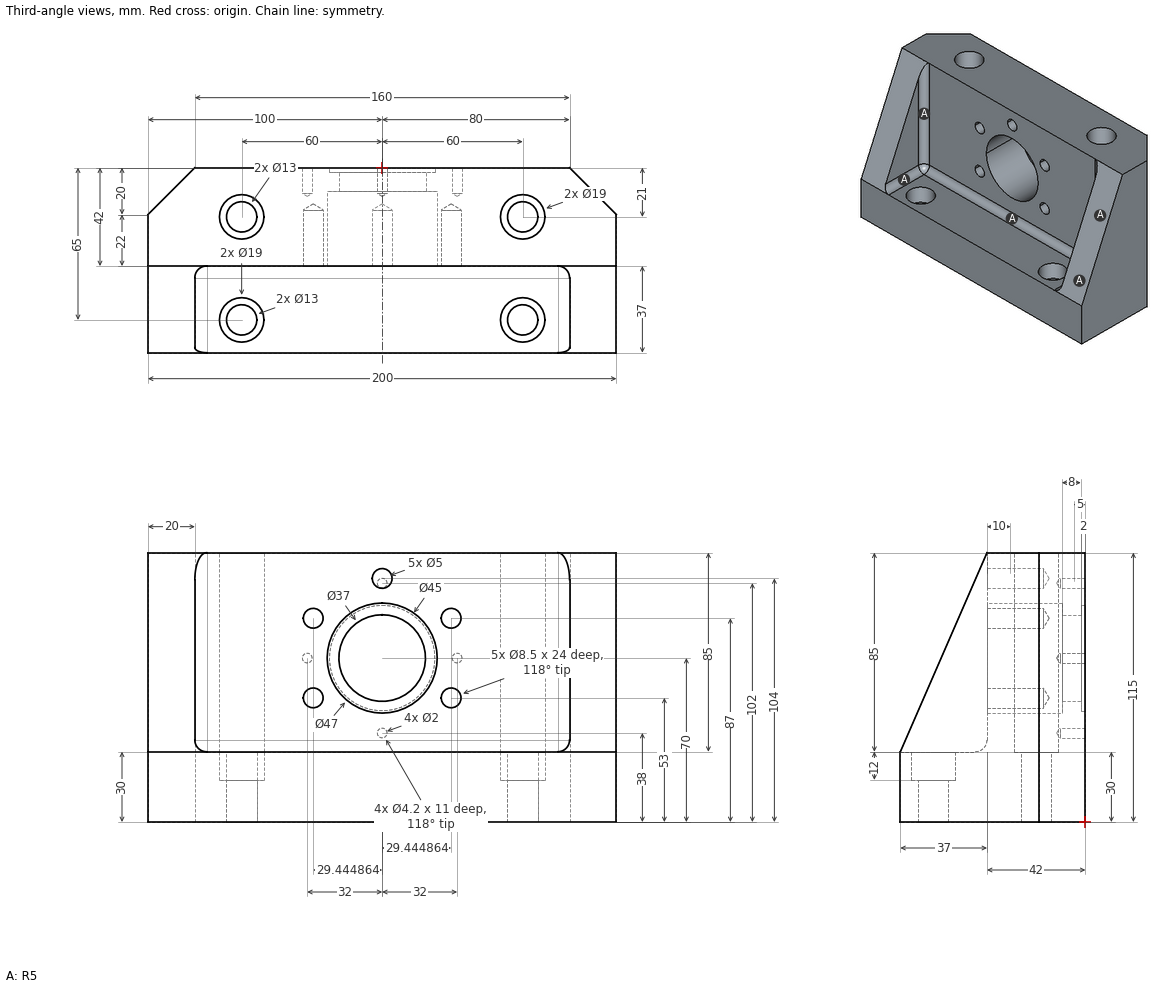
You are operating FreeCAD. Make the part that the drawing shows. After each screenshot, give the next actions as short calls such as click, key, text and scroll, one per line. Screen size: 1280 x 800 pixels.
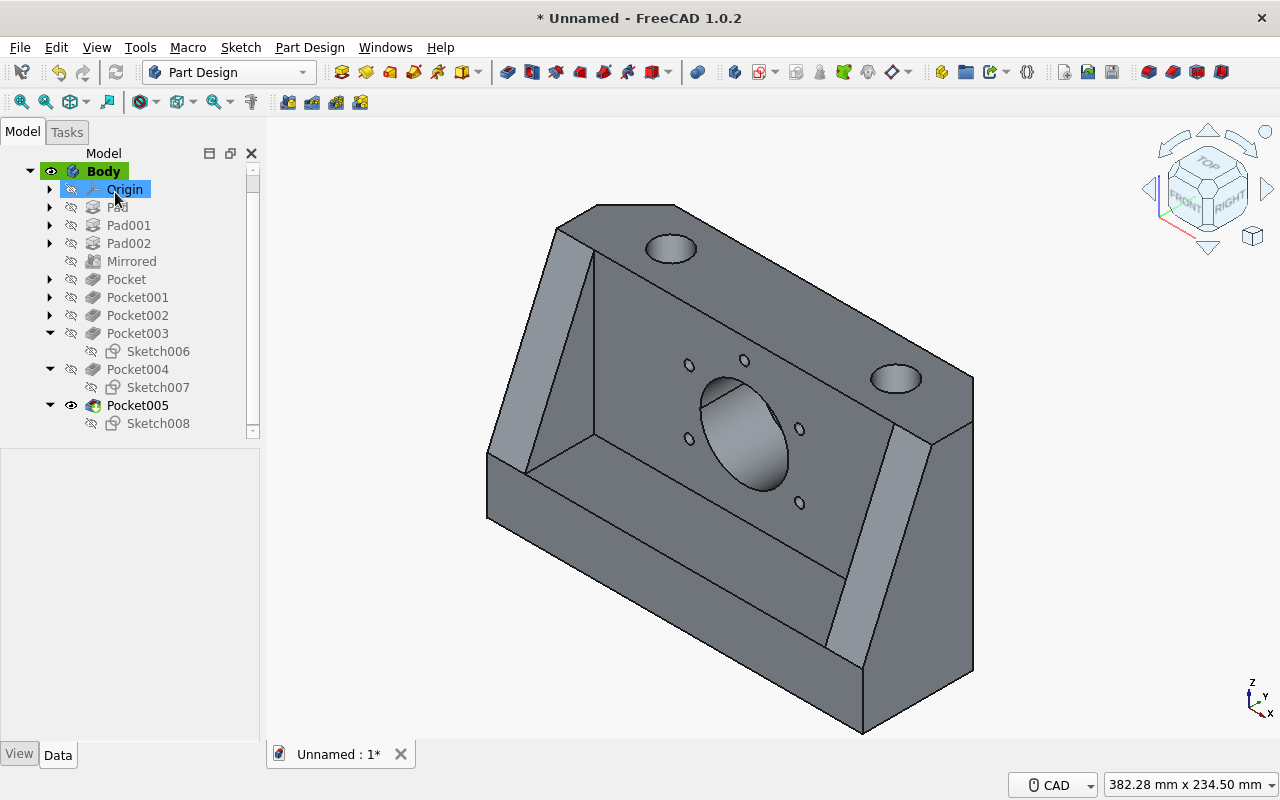
key(2)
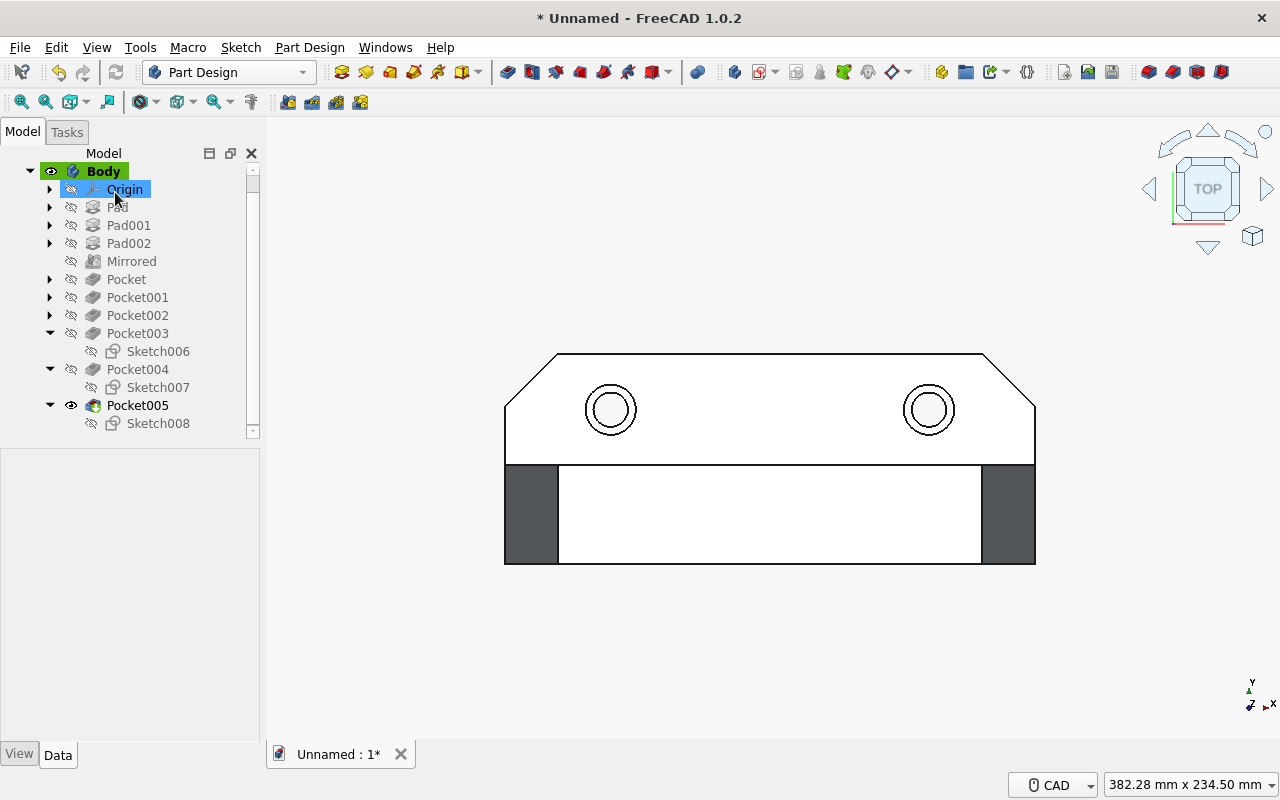
key(0)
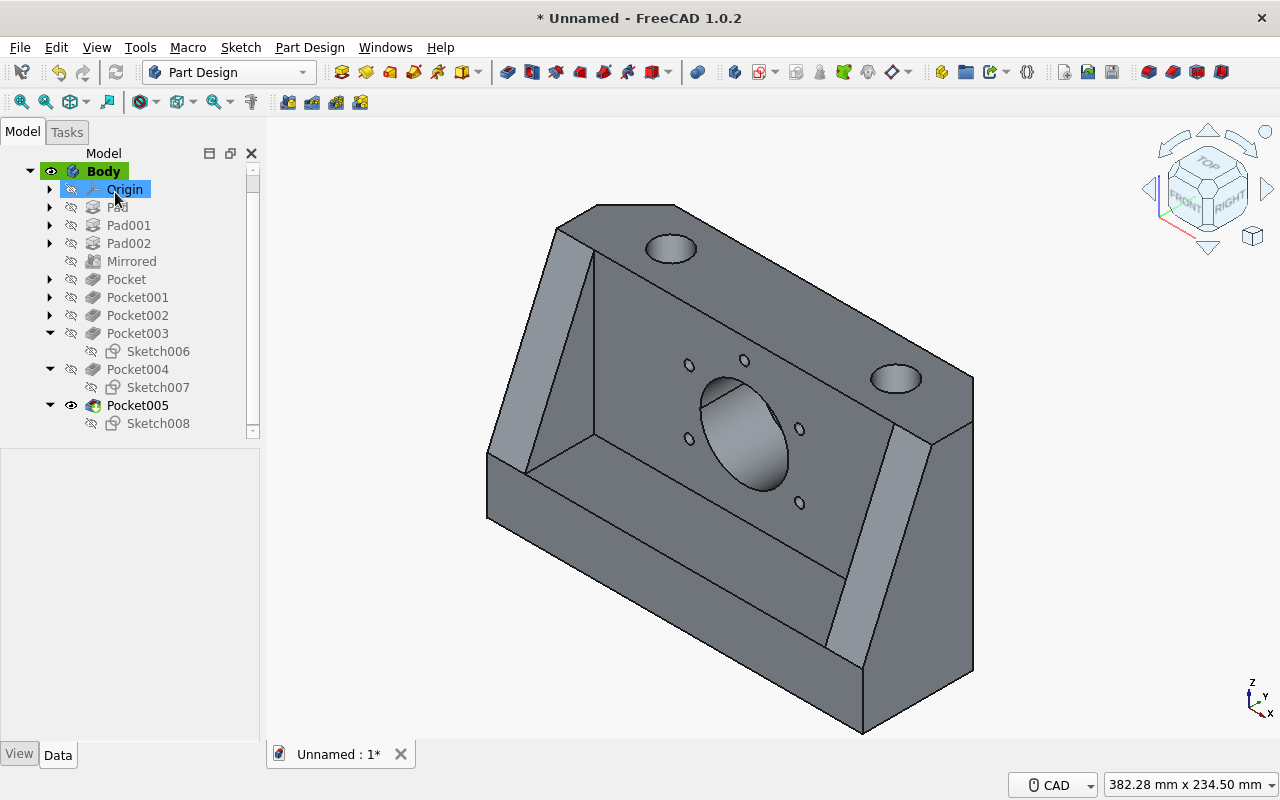
key(1)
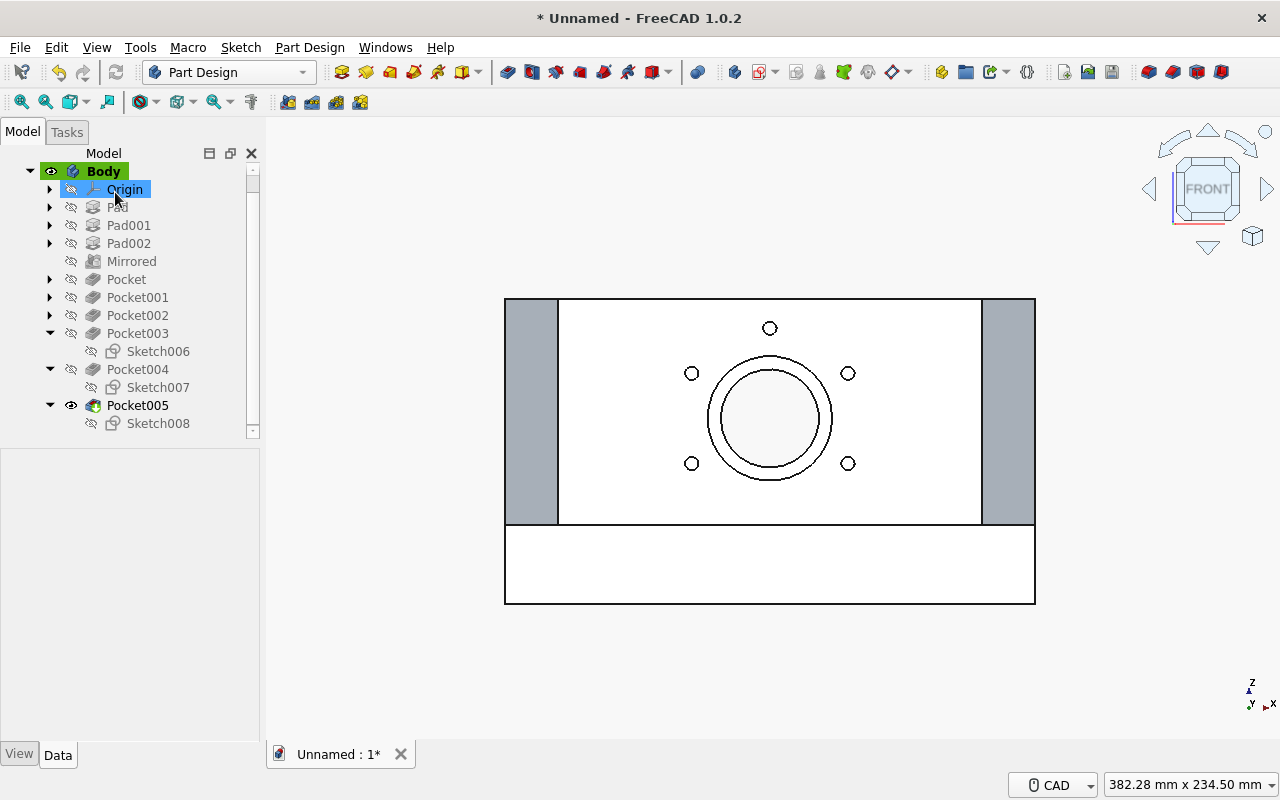
key(3)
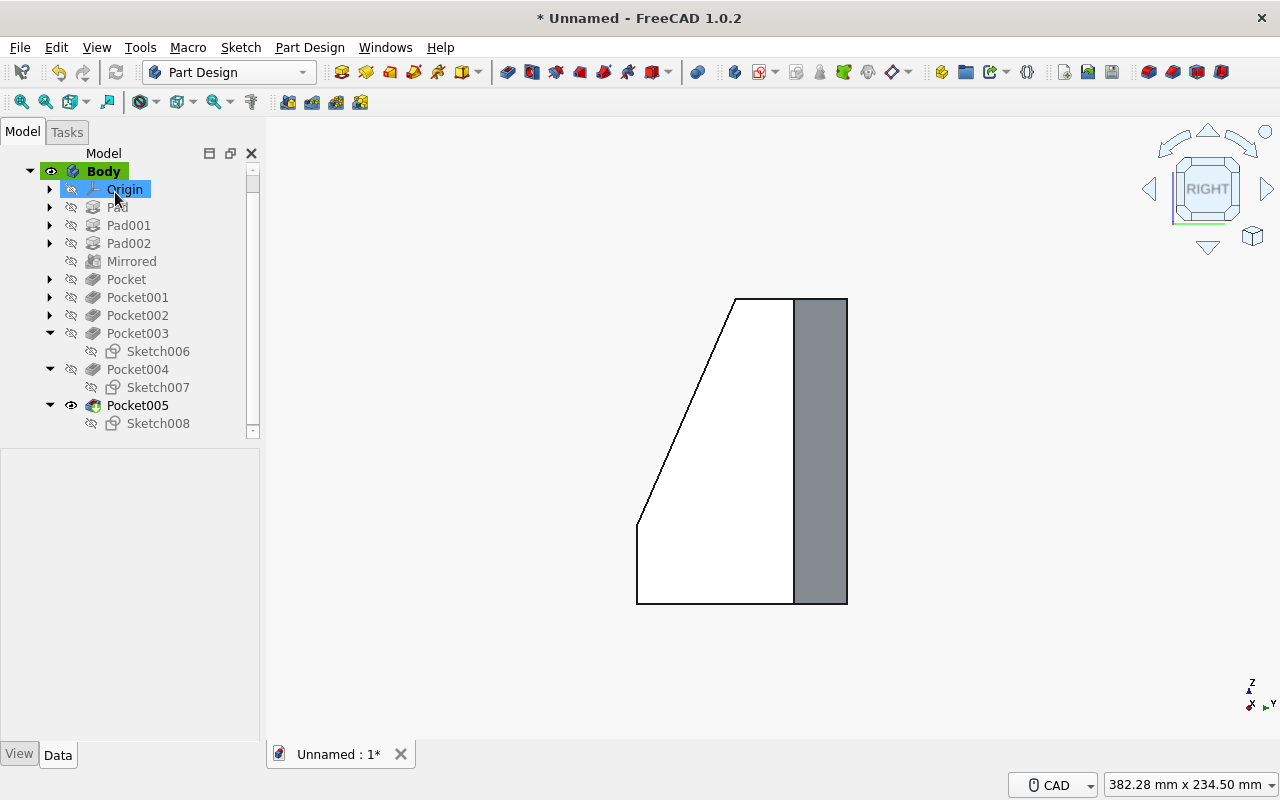
key(5)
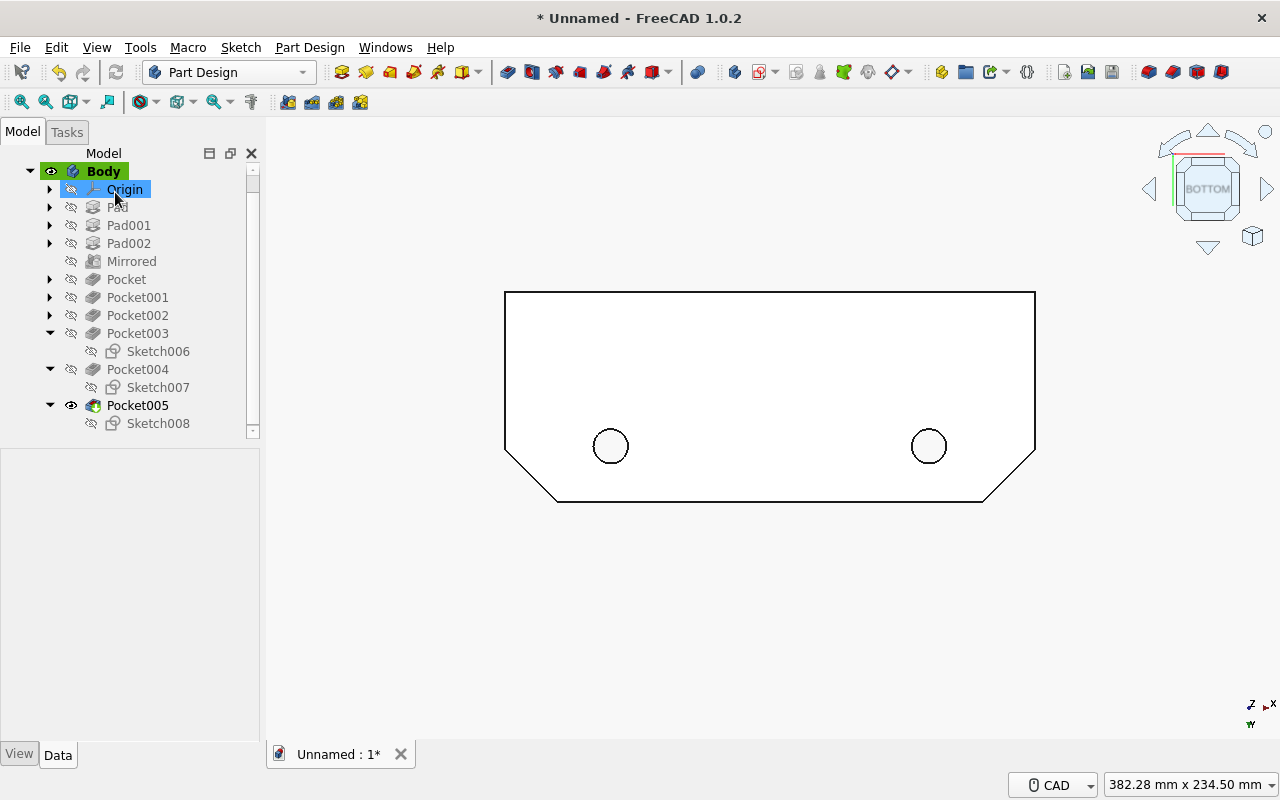
key(4)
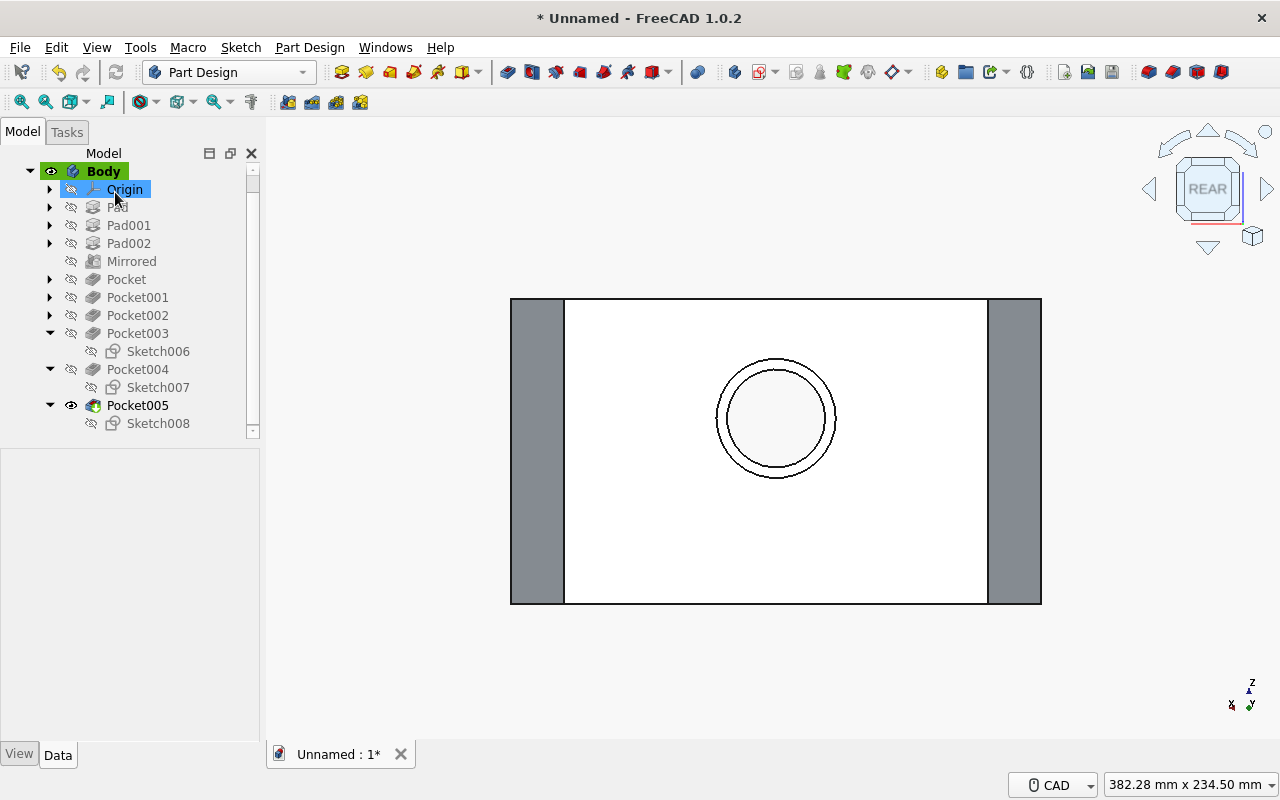
key(6)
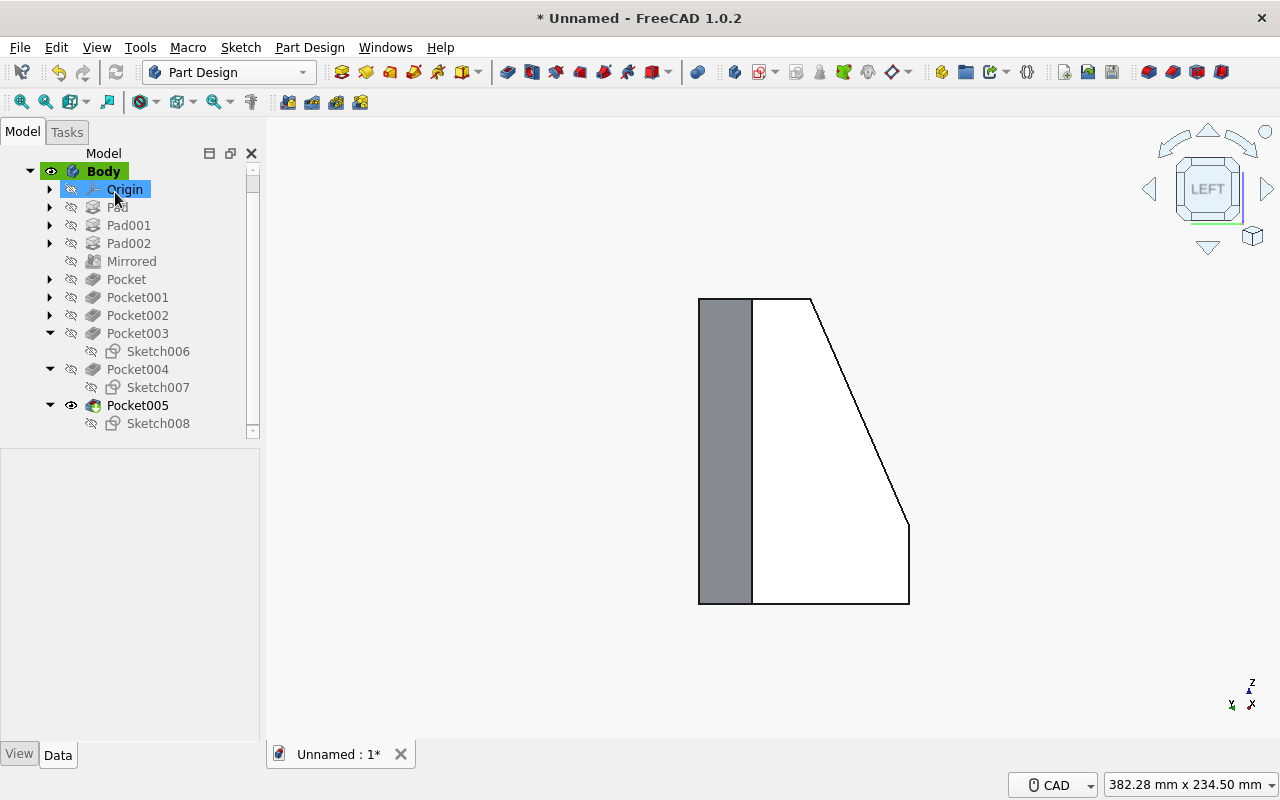
key(v)
key(3)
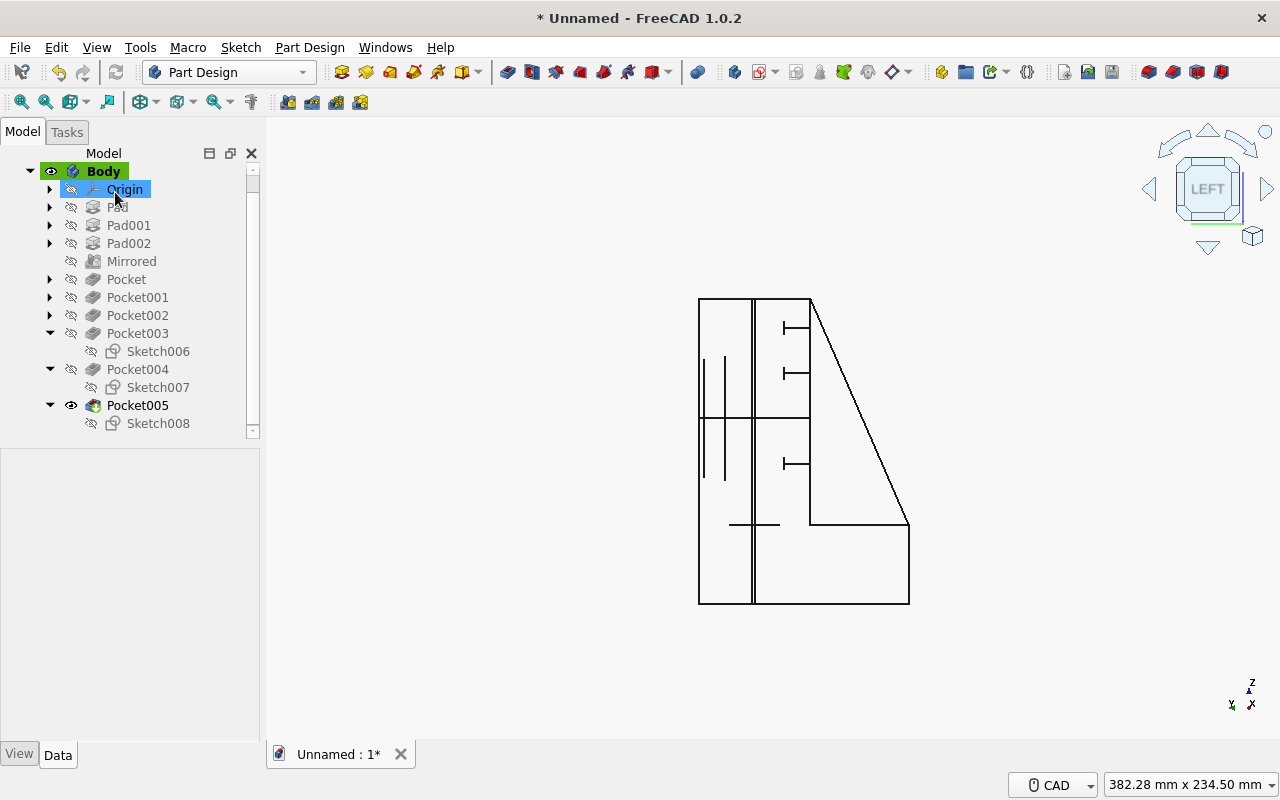
key(0)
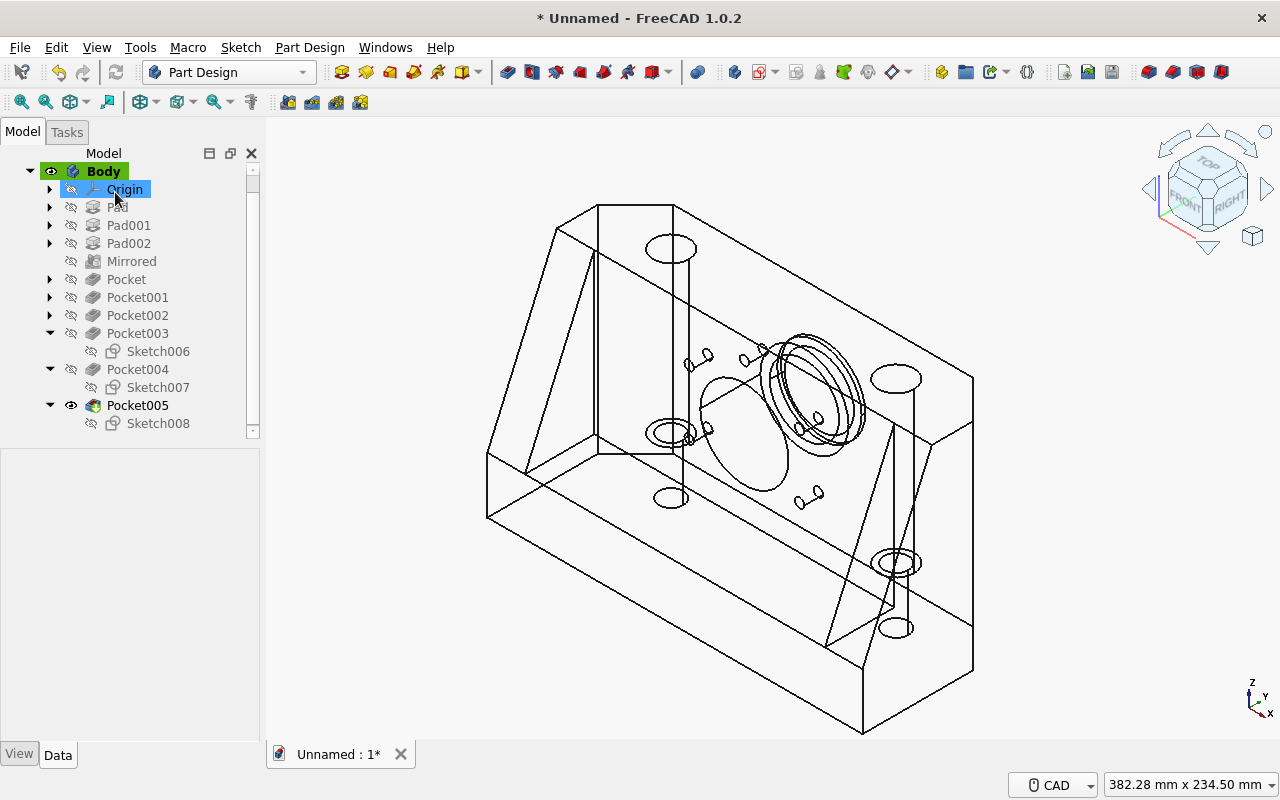
click(560, 453)